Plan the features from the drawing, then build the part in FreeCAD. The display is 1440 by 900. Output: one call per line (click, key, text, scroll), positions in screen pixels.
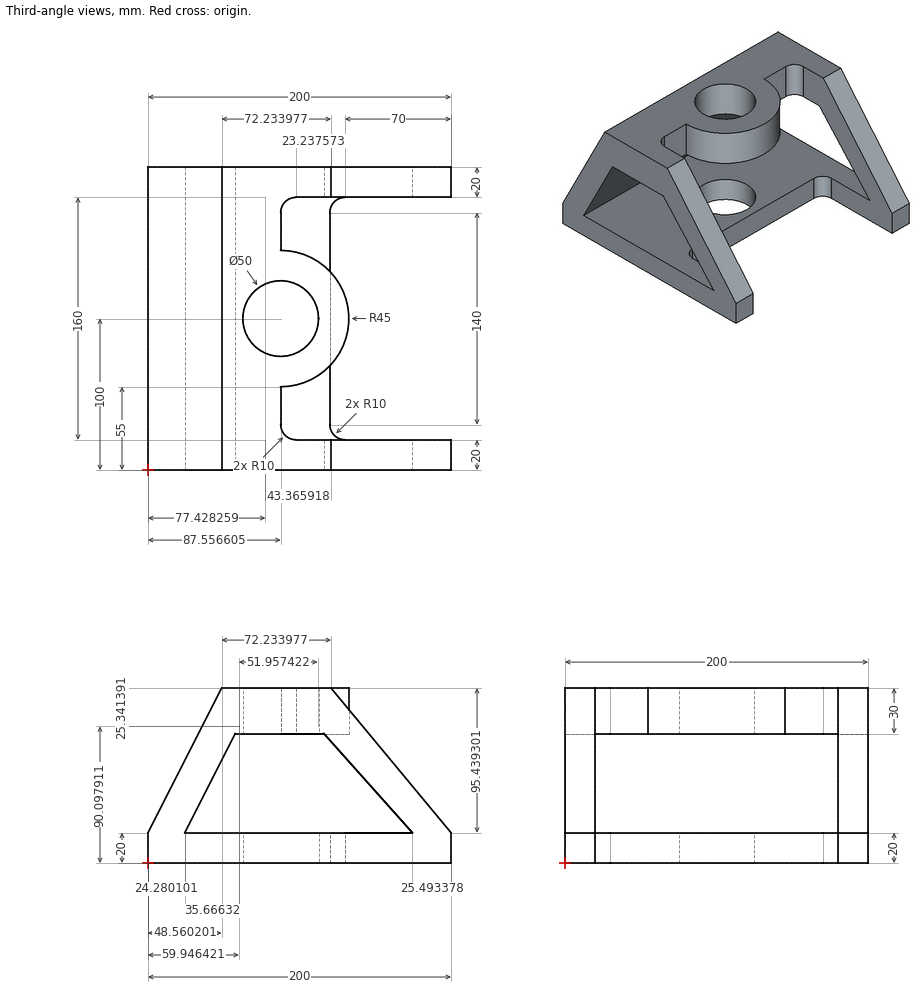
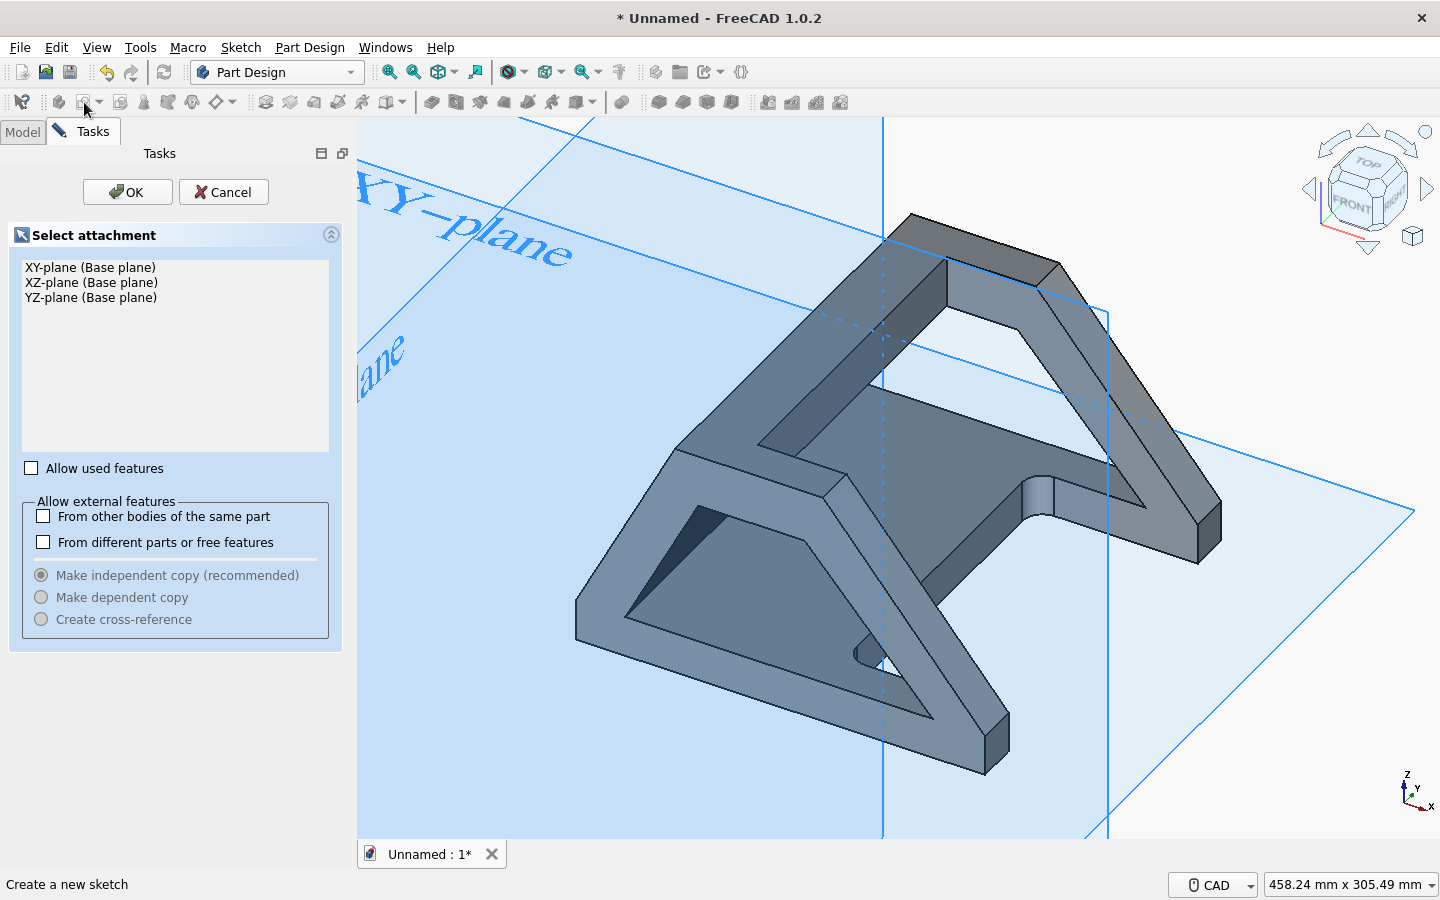
click(82, 282)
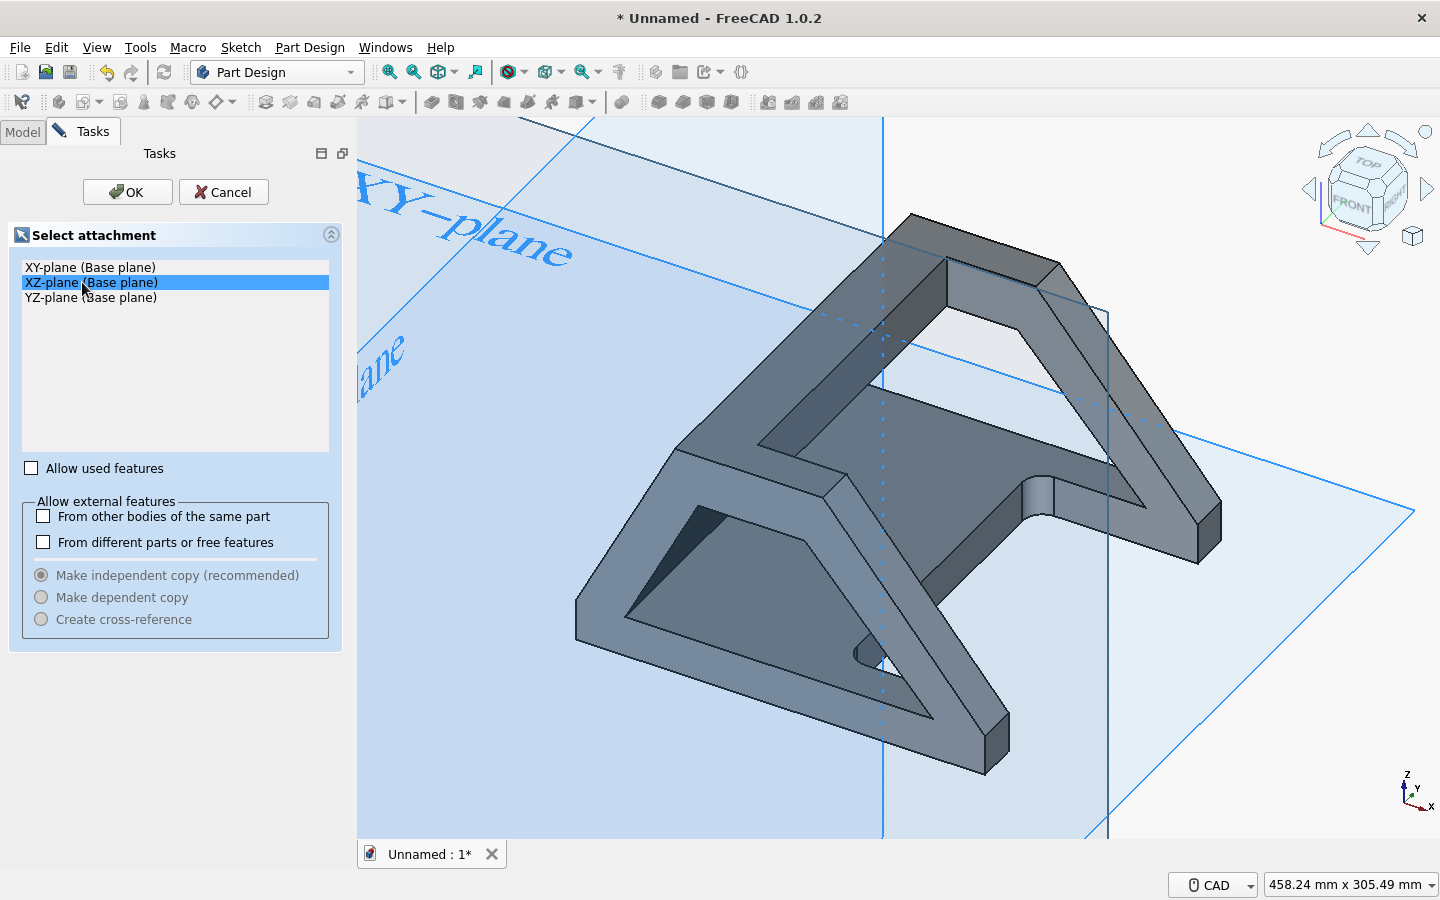
click(128, 192)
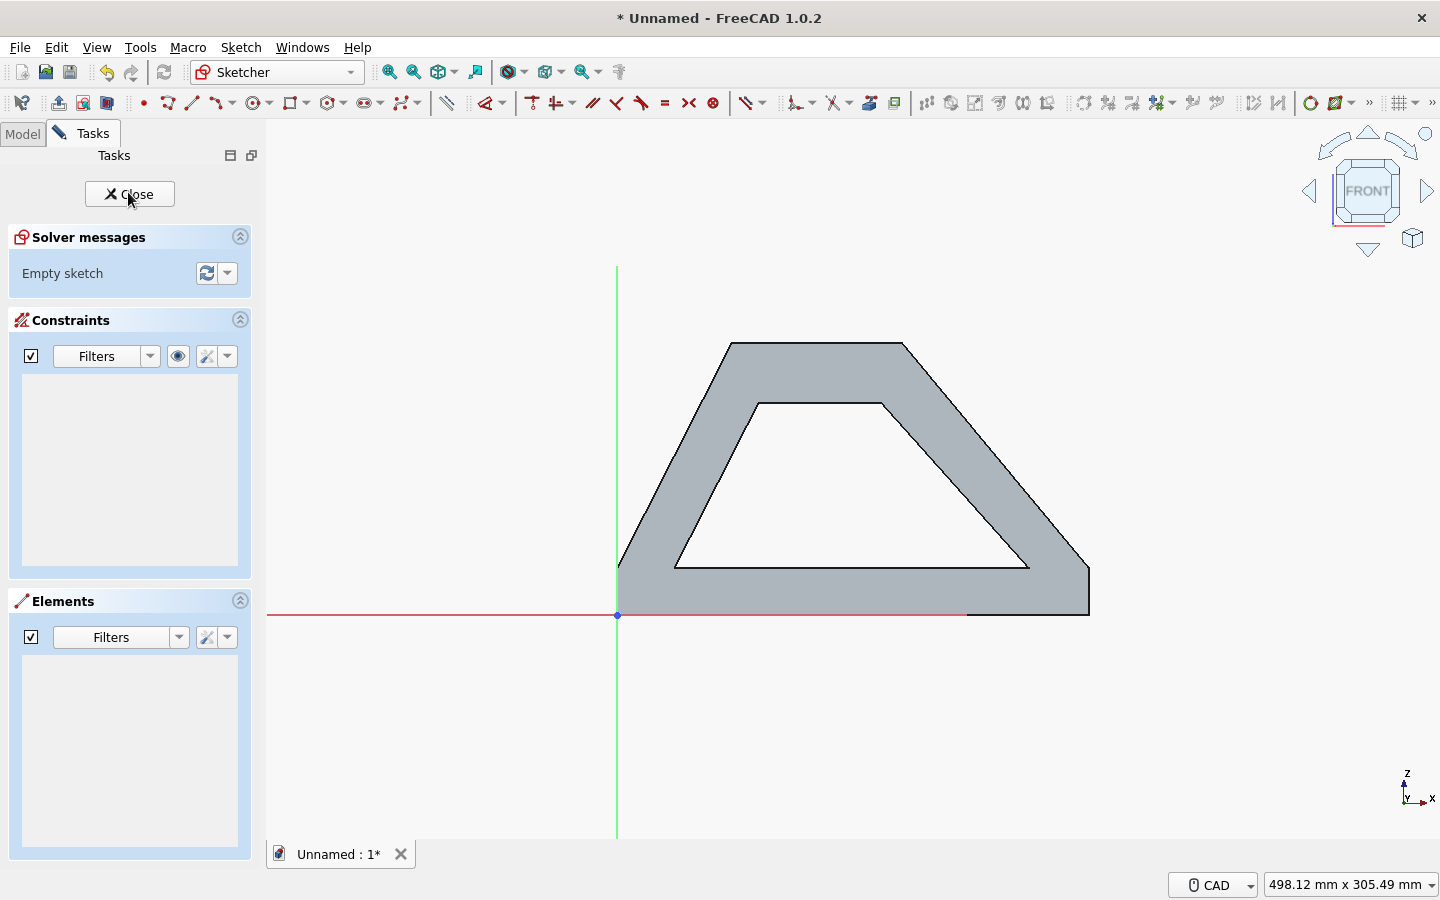
scroll(706, 479, up, 3)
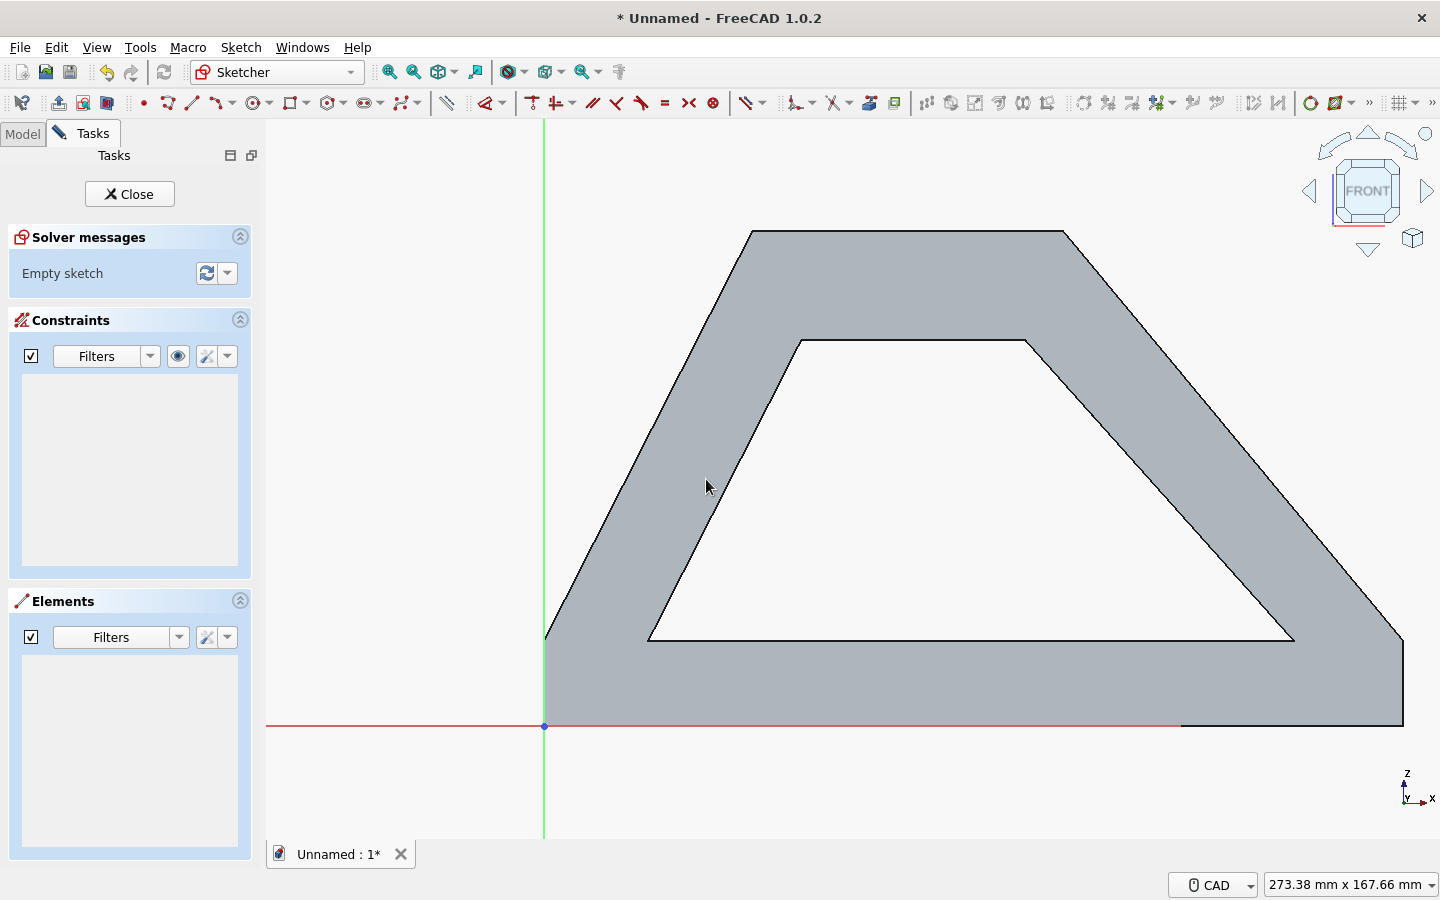
click(290, 104)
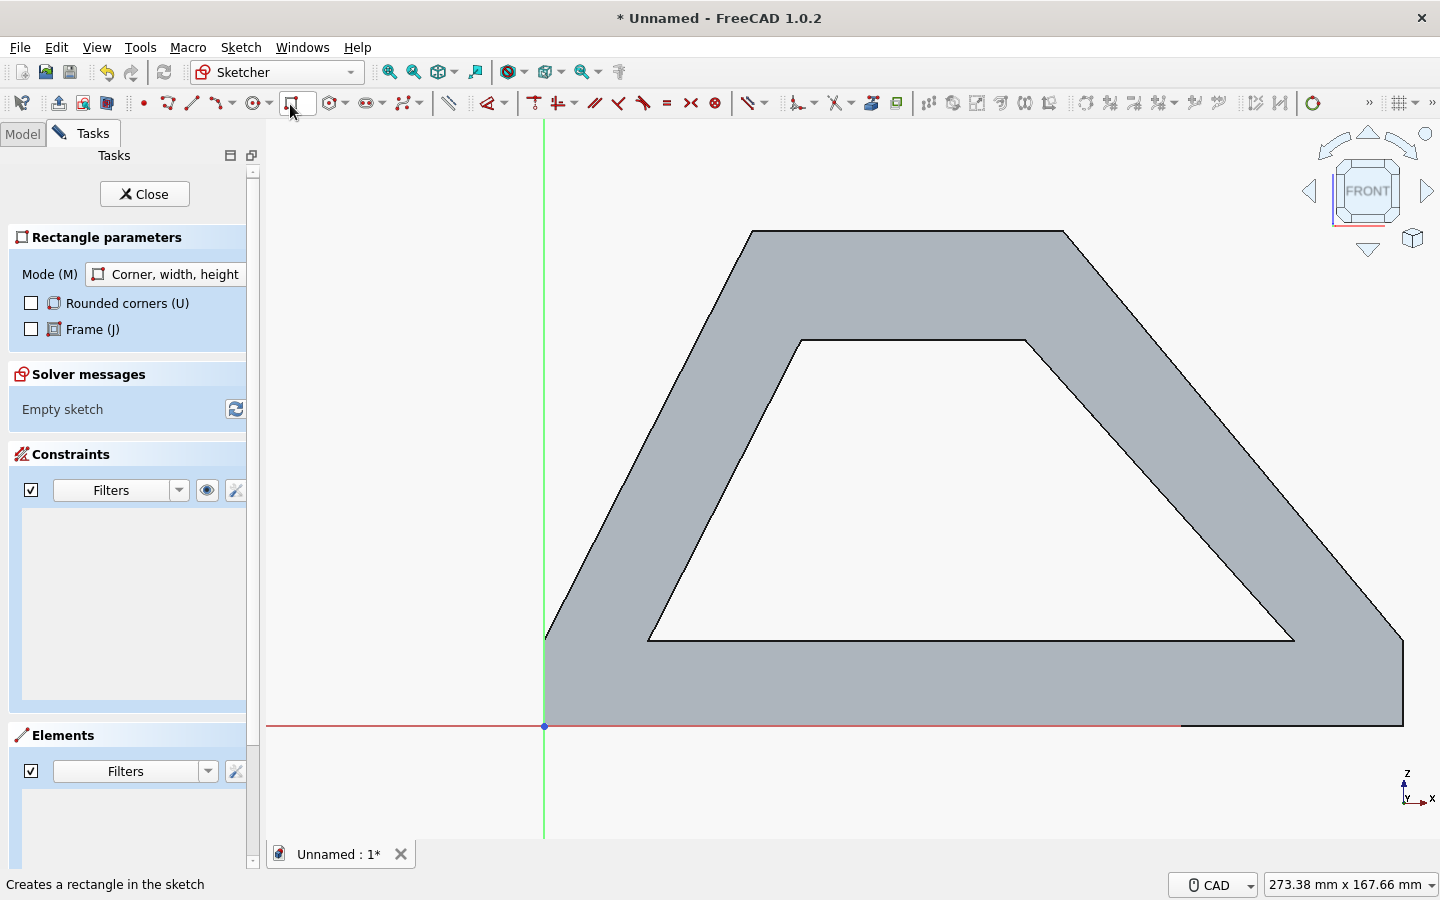
click(802, 231)
click(1025, 340)
key(Escape)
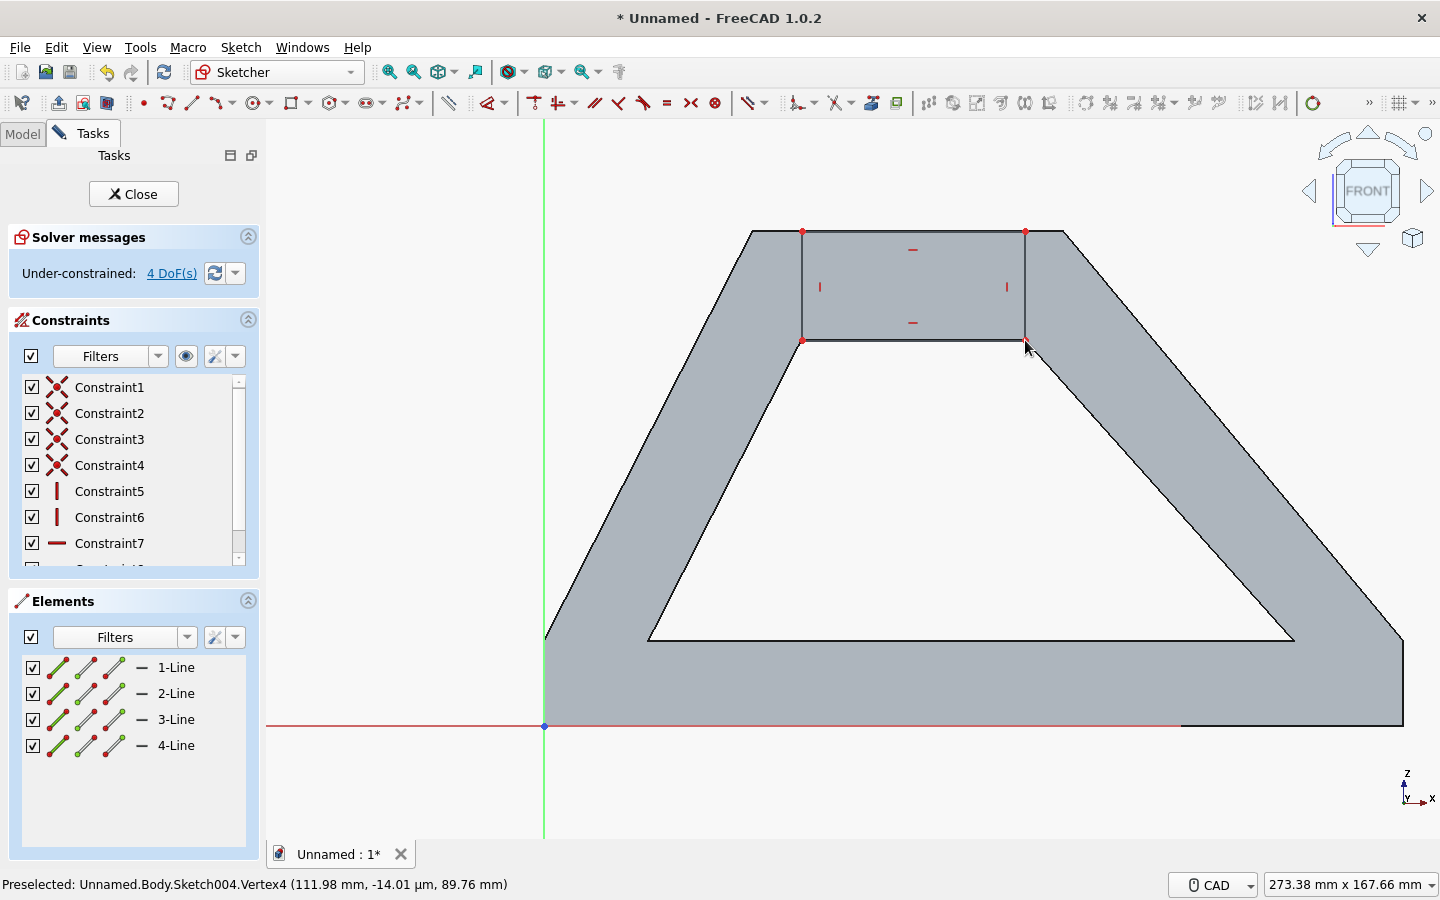
click(488, 104)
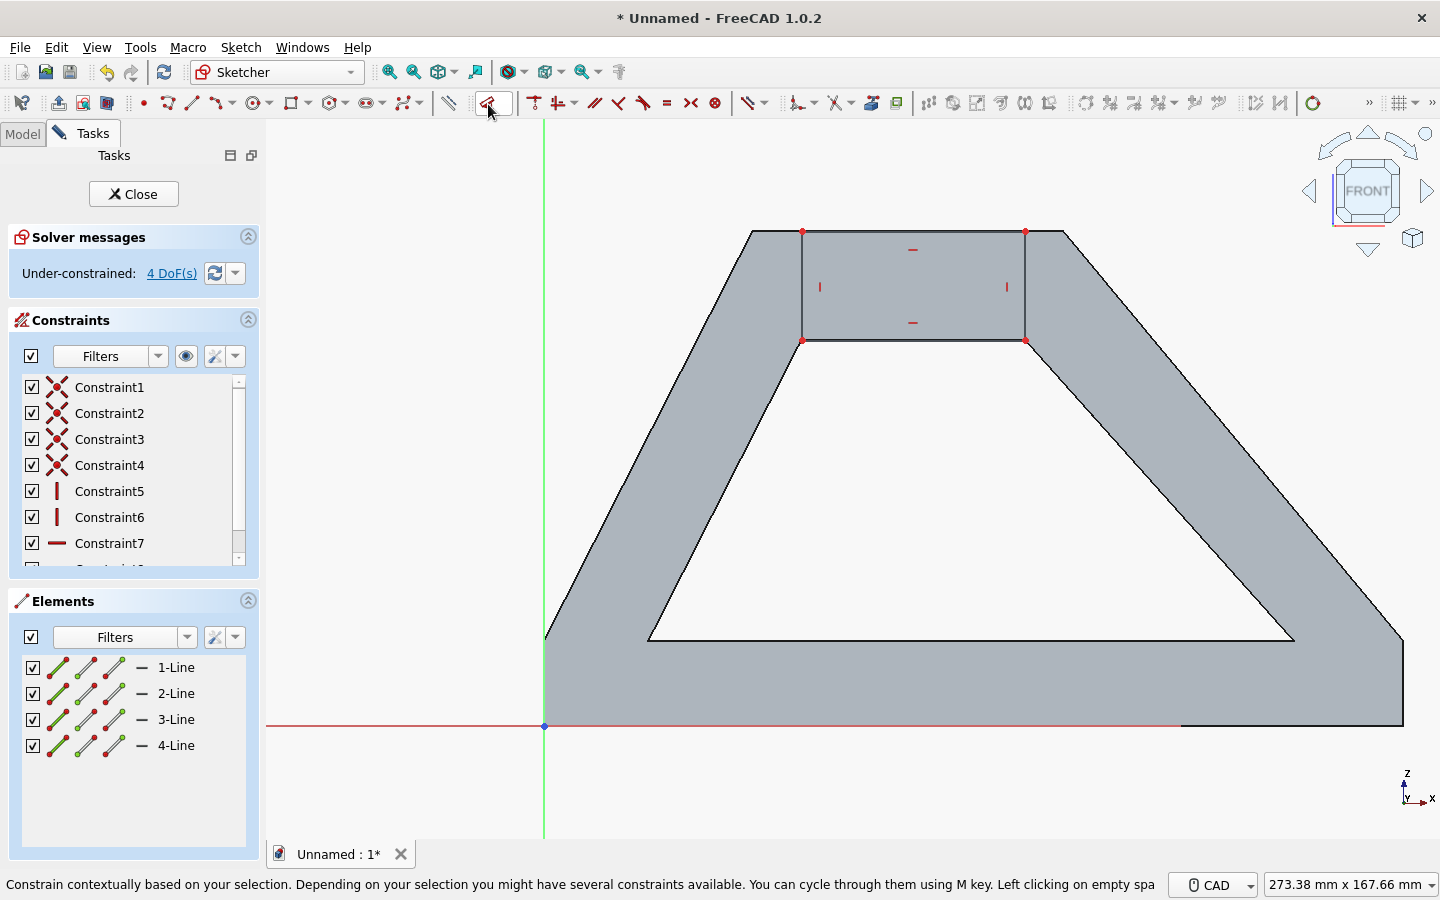
click(802, 265)
click(836, 287)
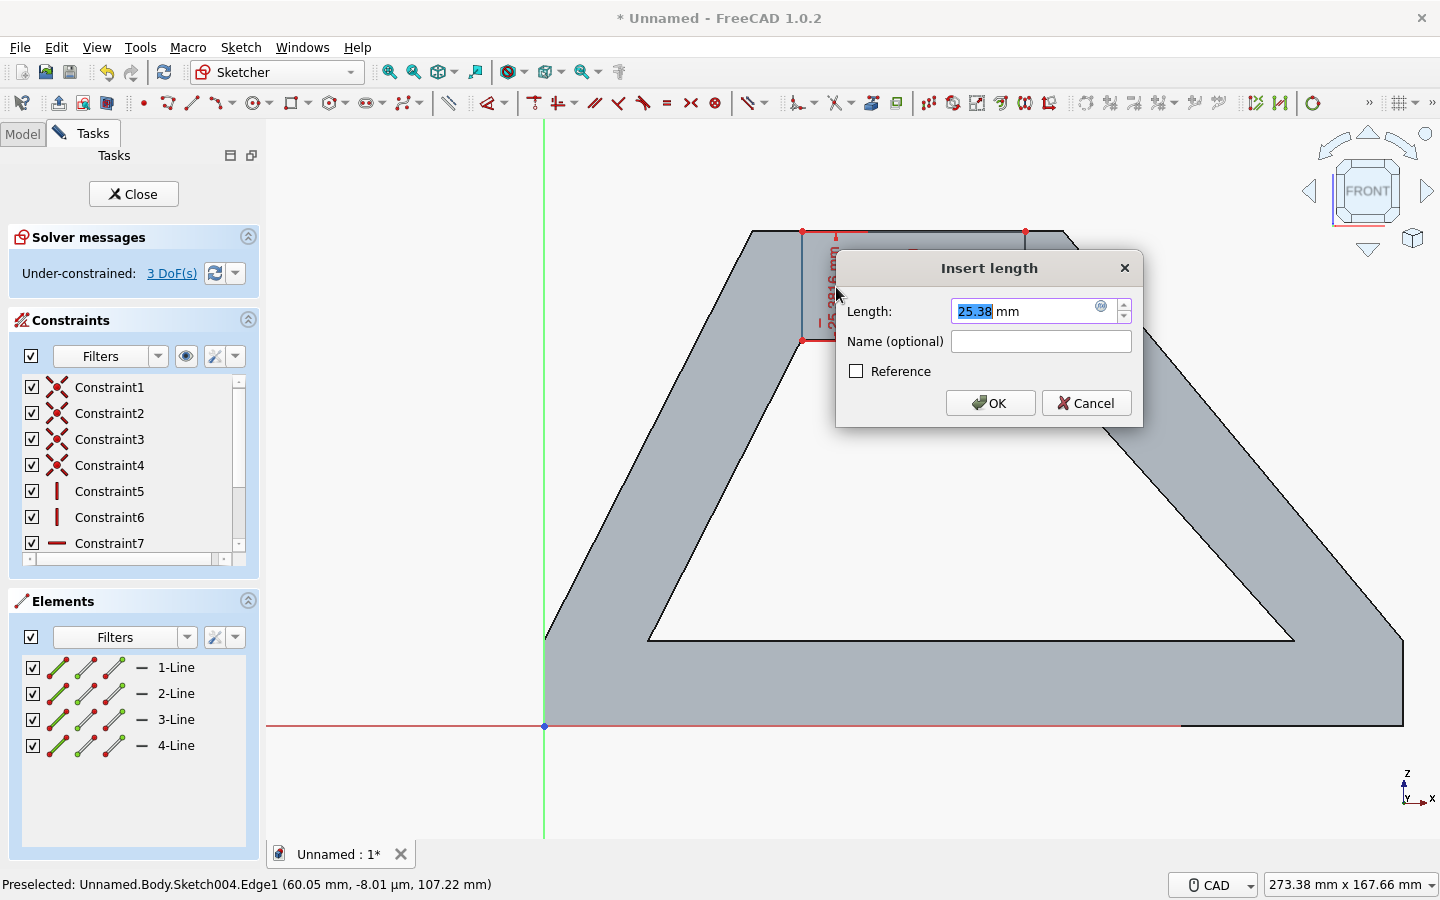
text(25.341391)
key(Return)